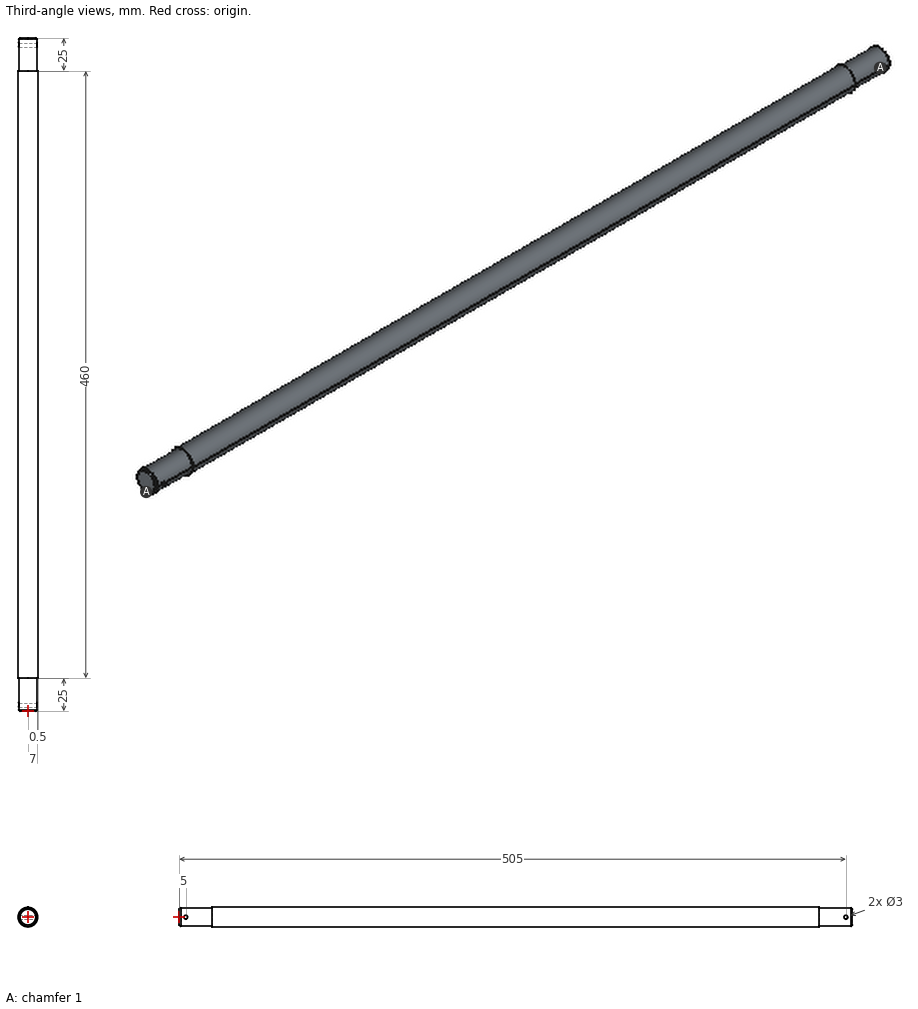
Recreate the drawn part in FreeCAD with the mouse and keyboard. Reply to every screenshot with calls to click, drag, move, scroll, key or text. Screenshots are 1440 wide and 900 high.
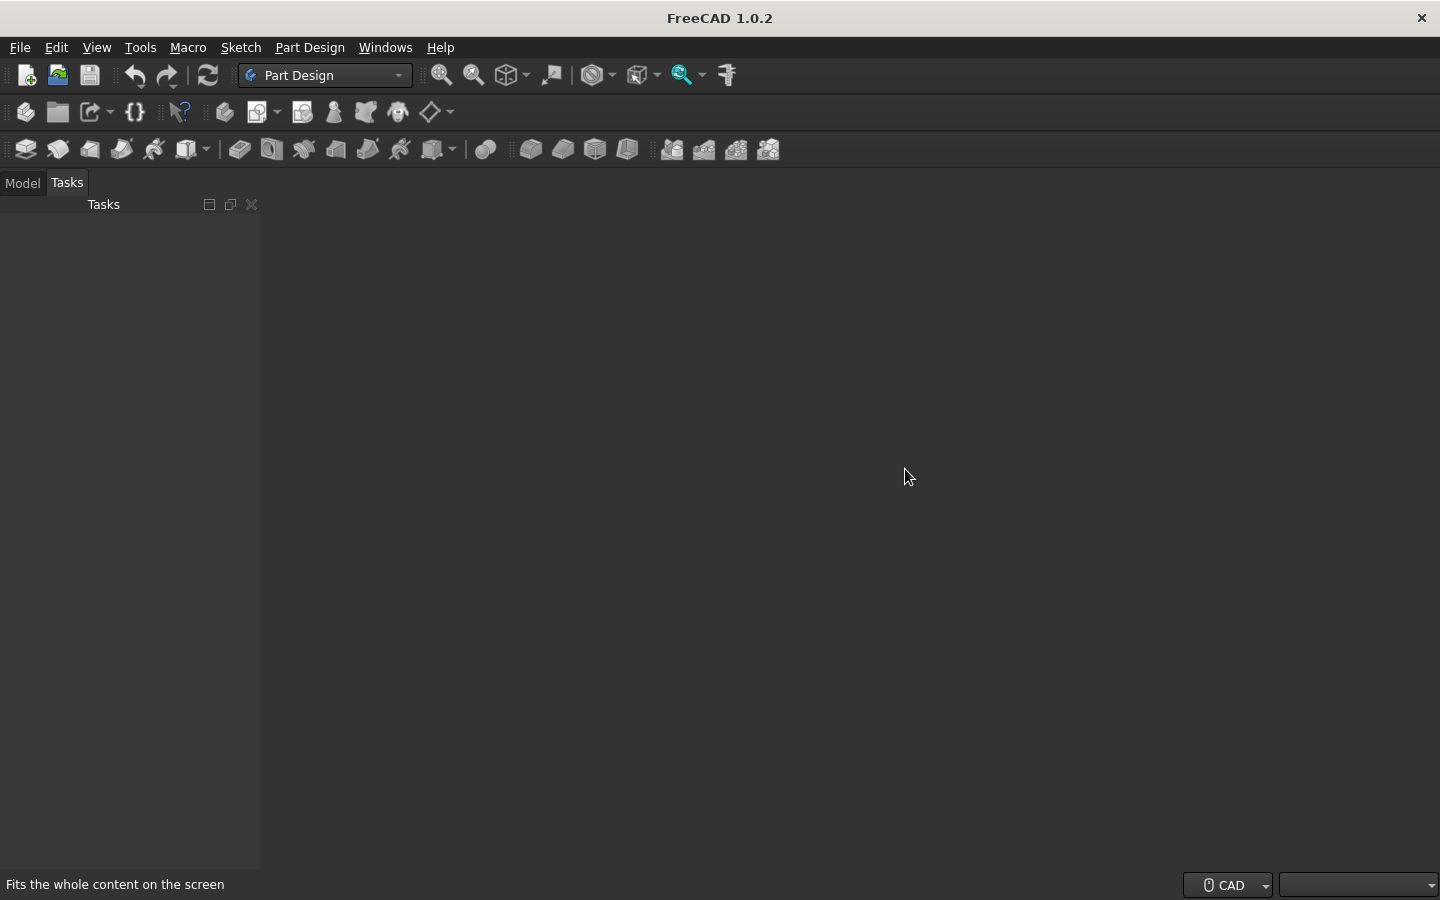
click(26, 76)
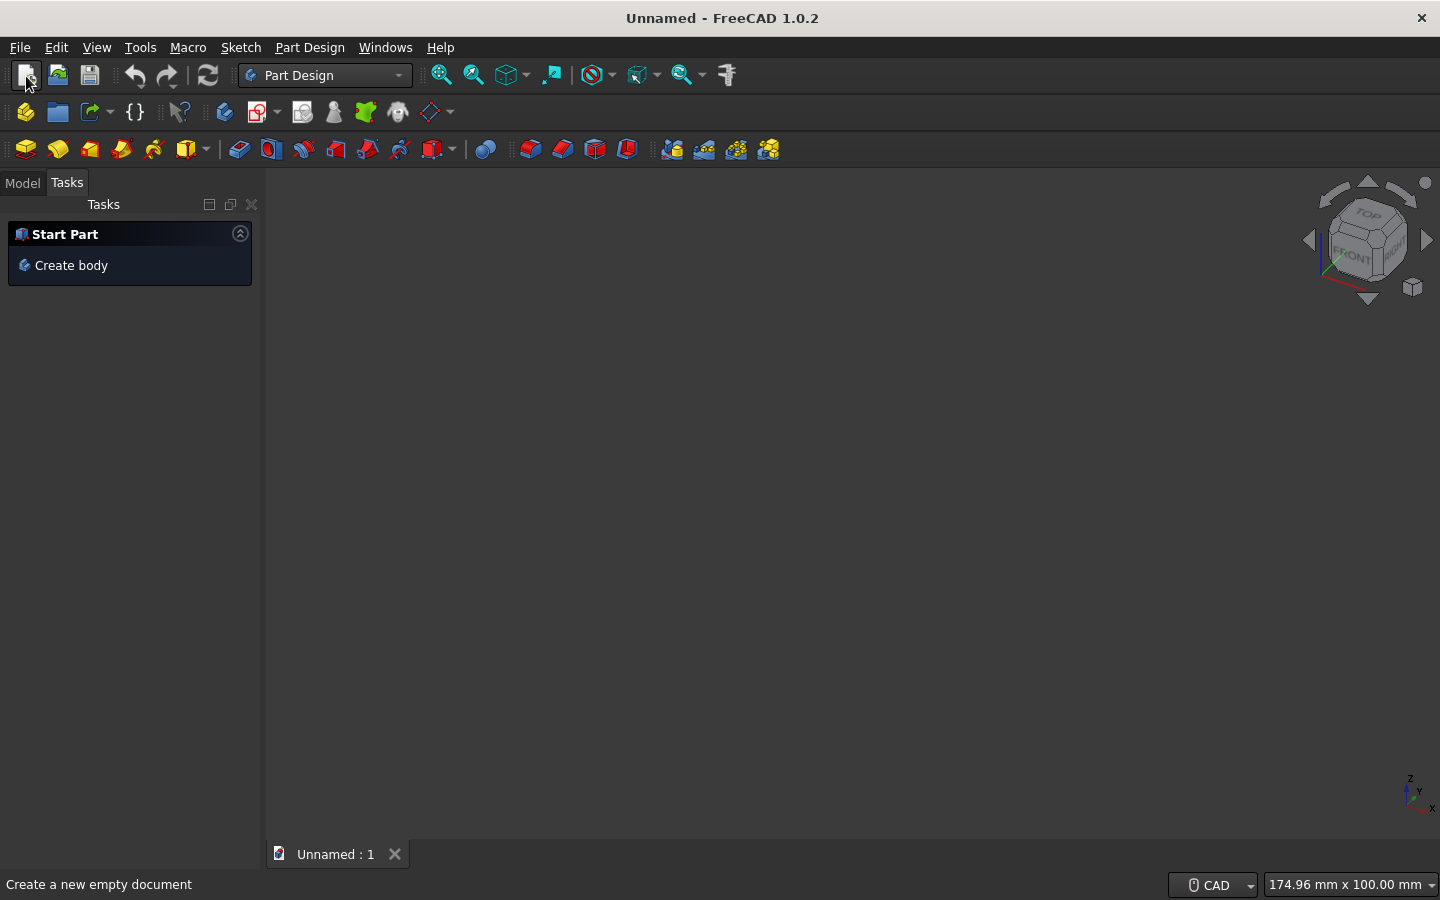
click(258, 112)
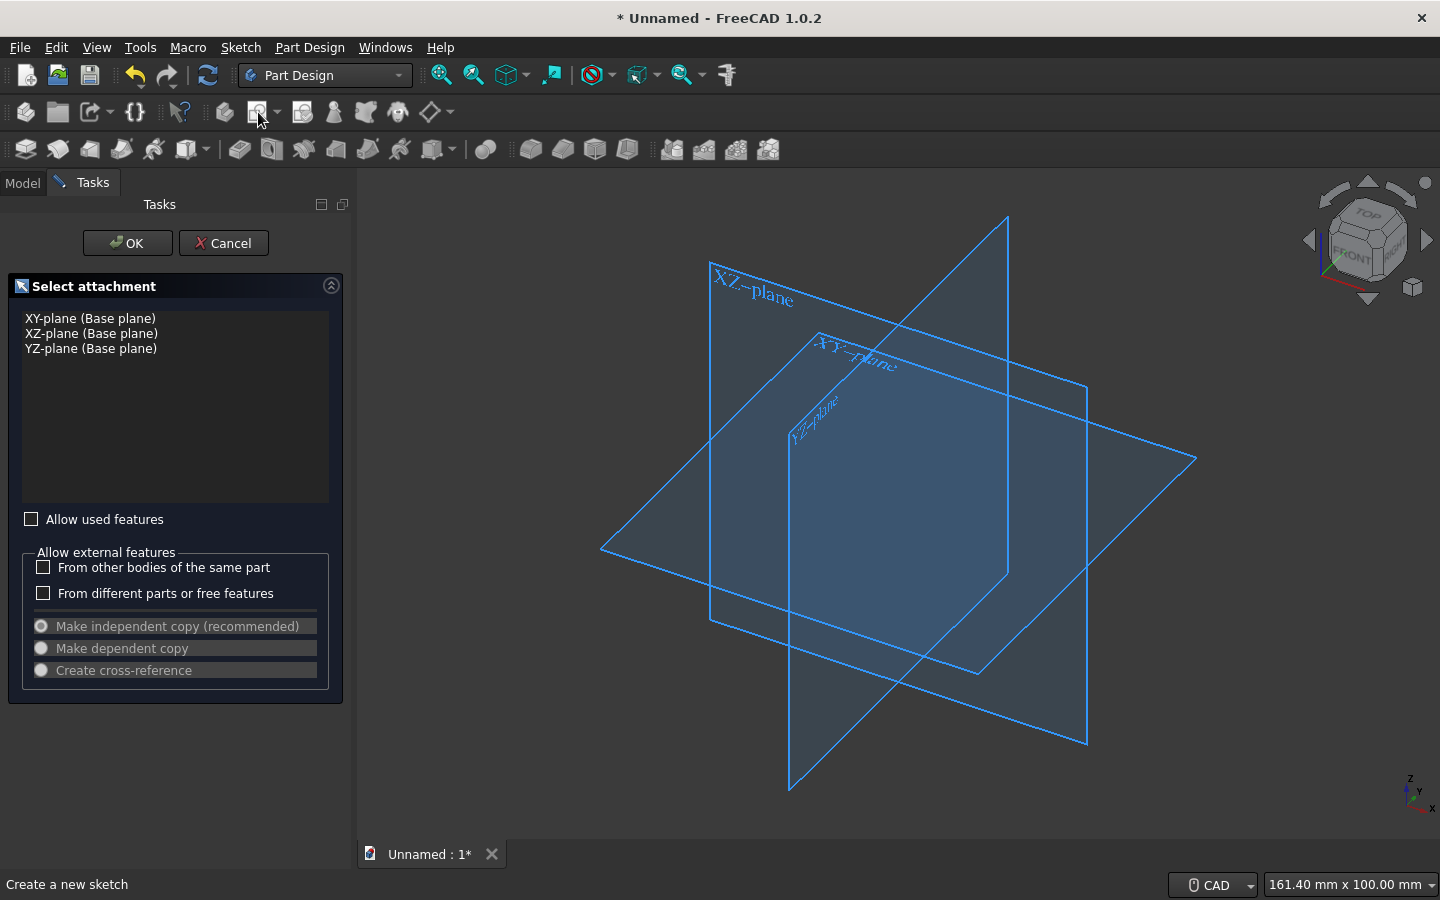
click(82, 318)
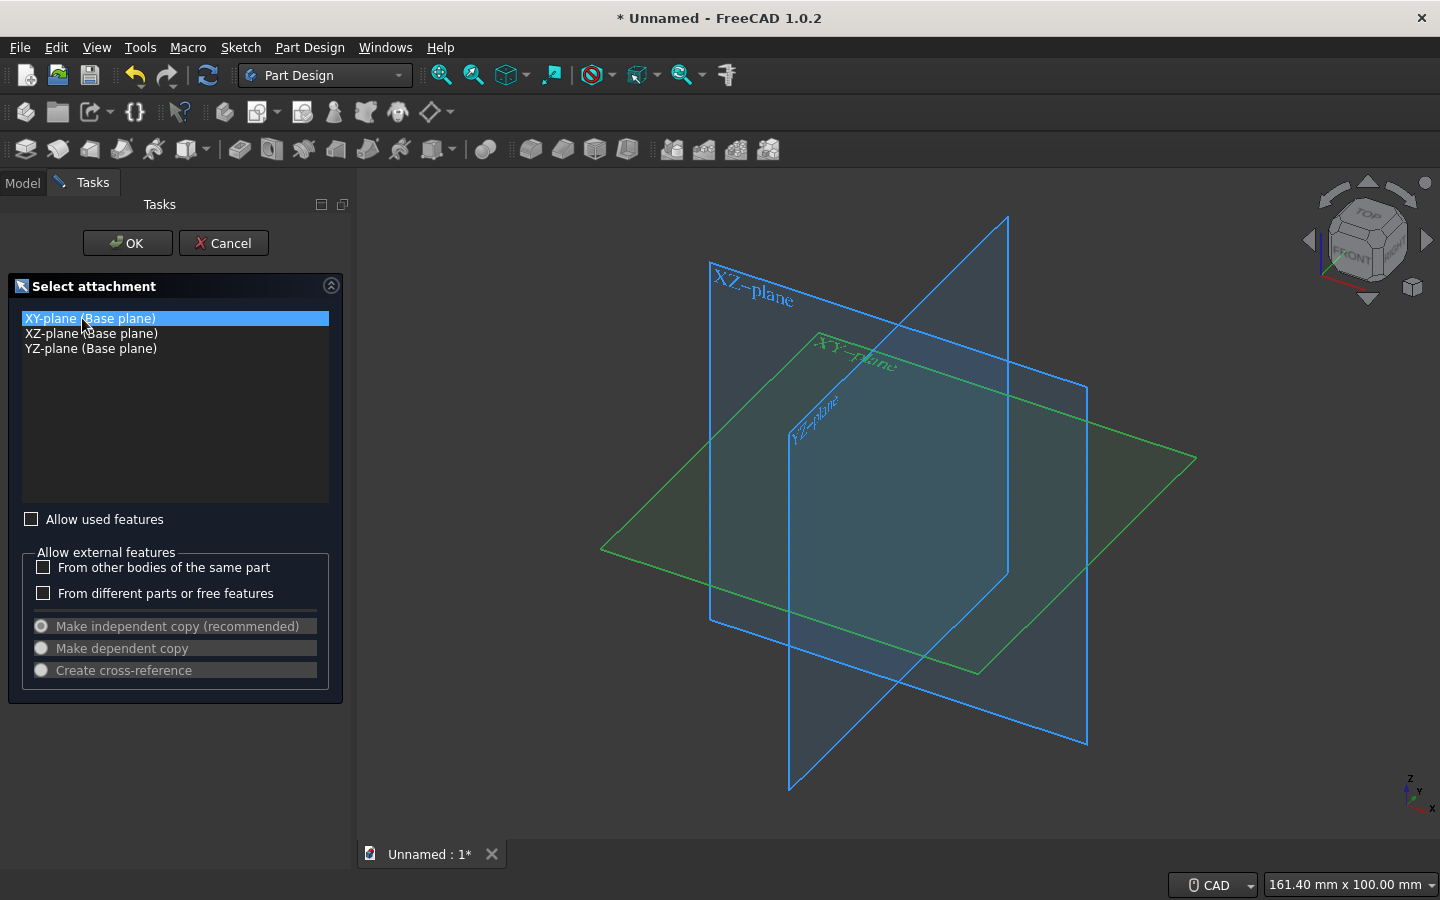
click(128, 243)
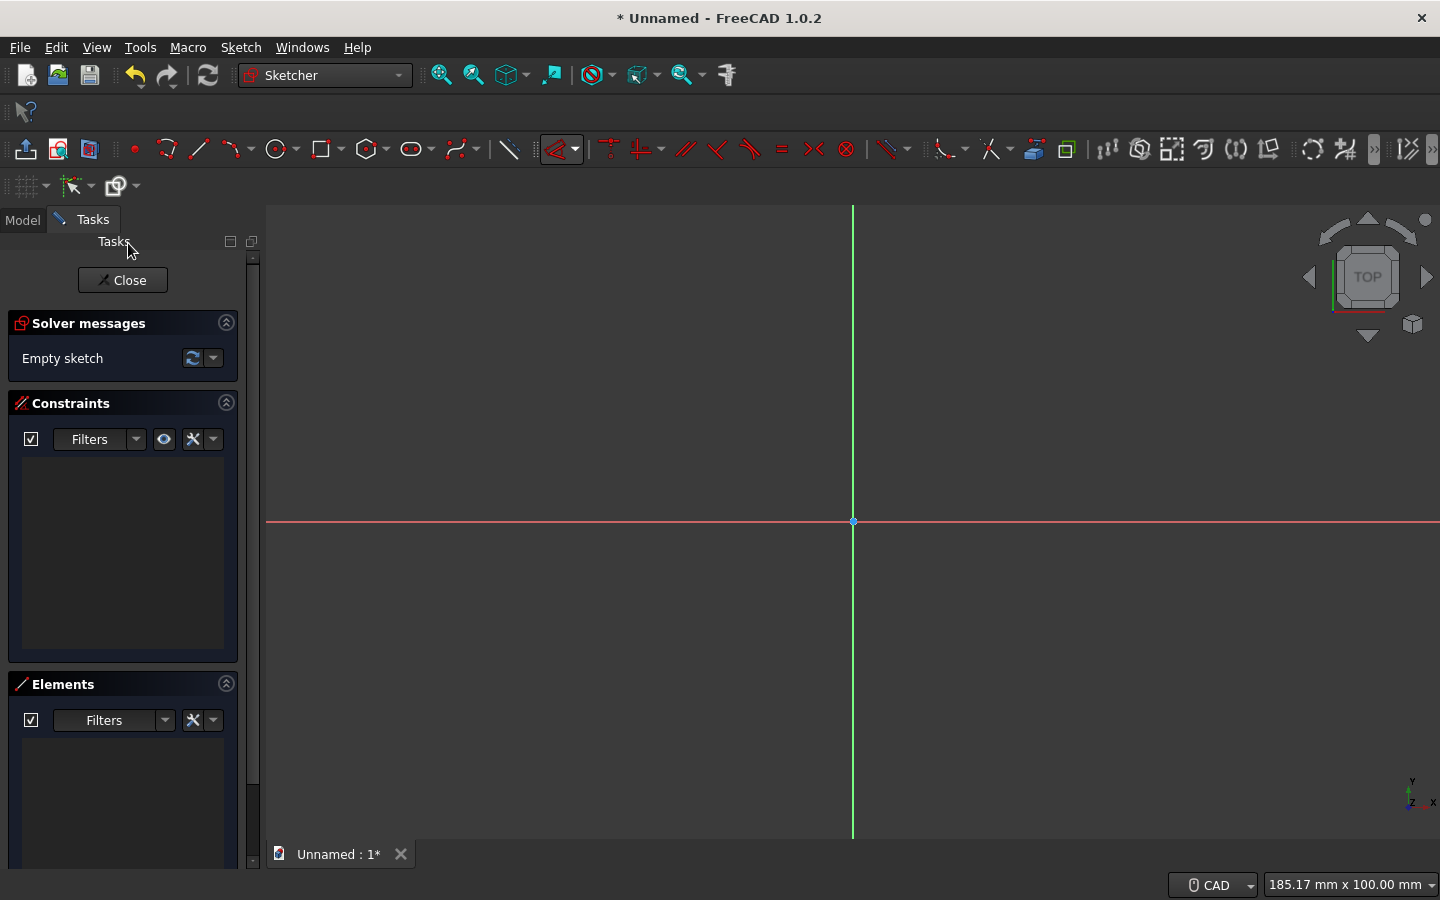
scroll(770, 775, down, 10)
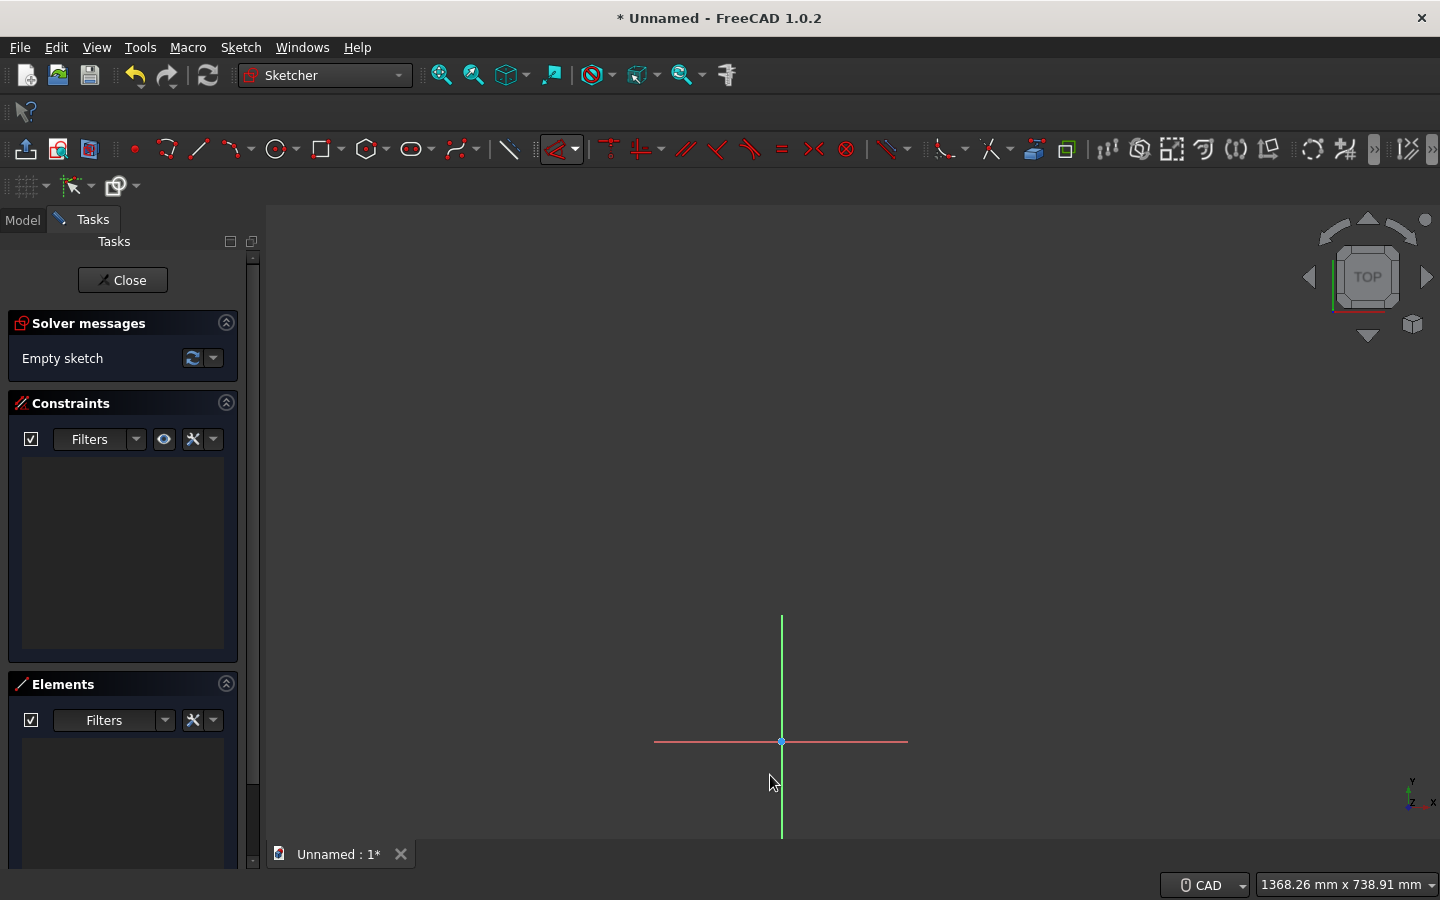
click(168, 150)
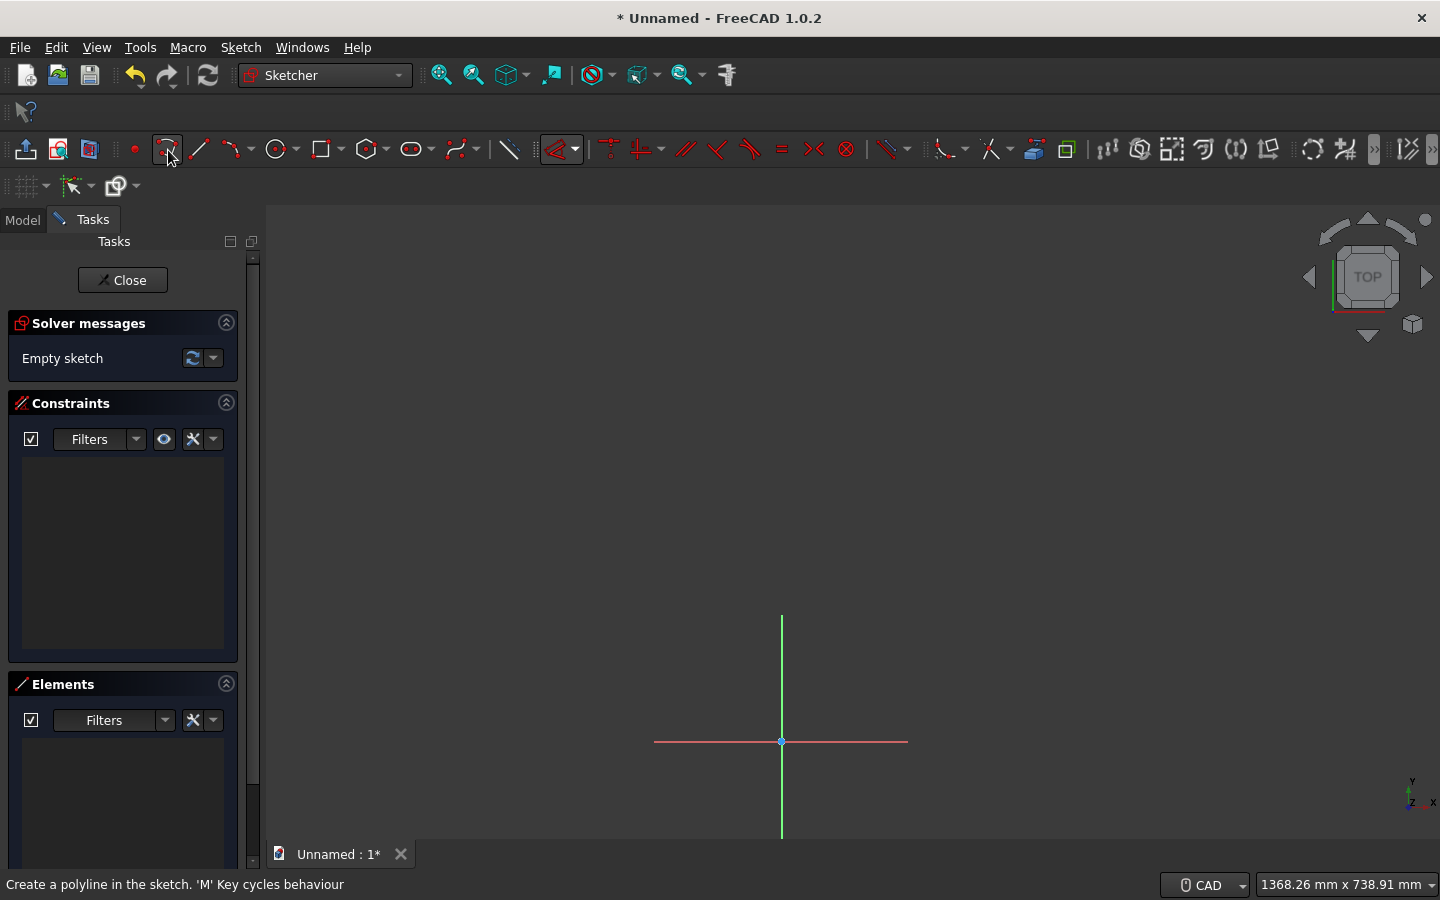
click(782, 742)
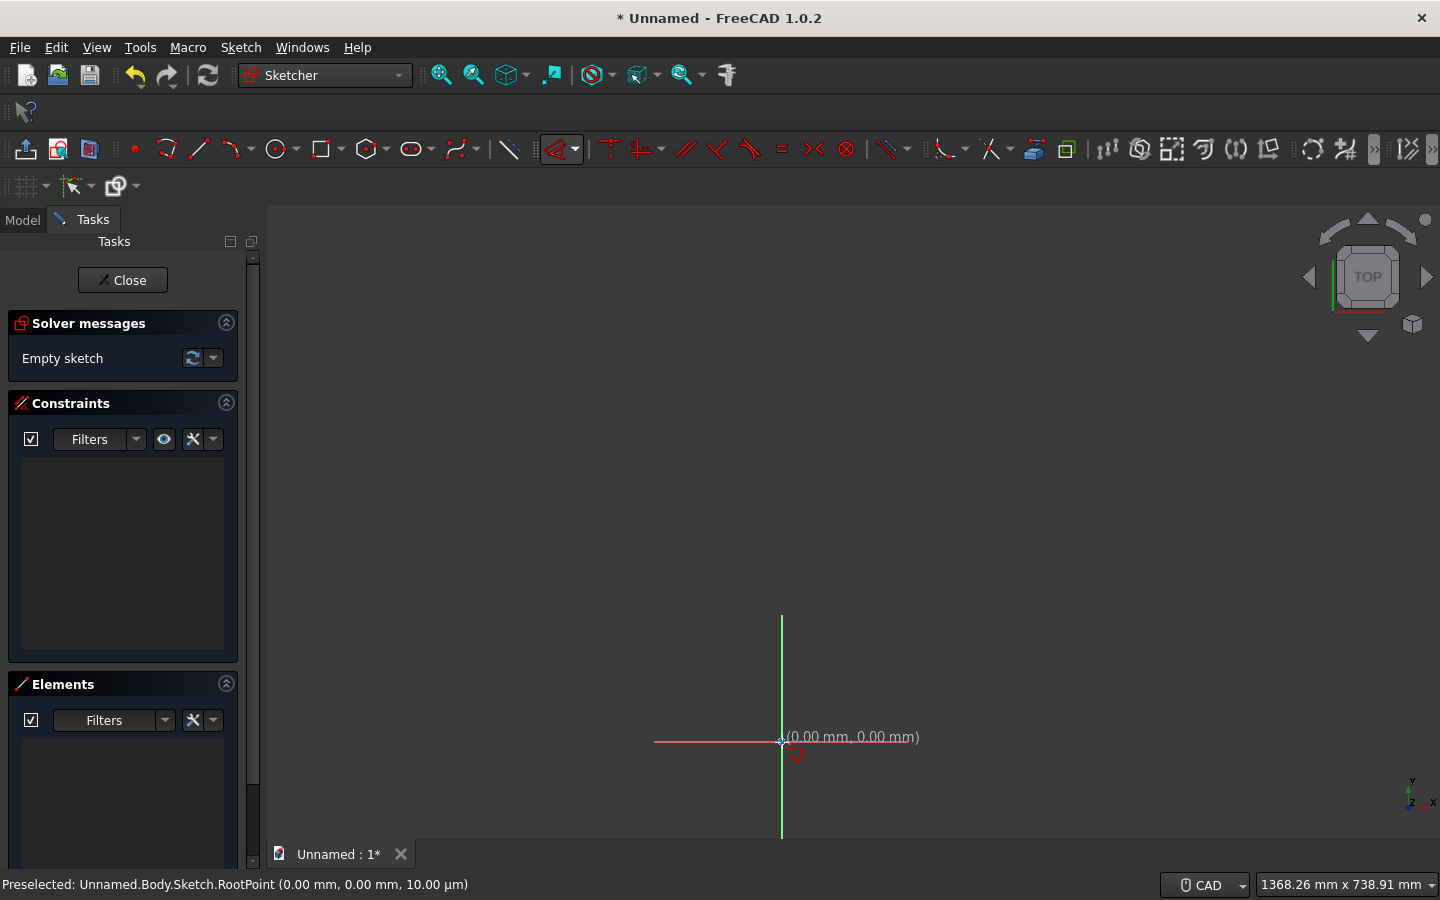
scroll(788, 742, up, 5)